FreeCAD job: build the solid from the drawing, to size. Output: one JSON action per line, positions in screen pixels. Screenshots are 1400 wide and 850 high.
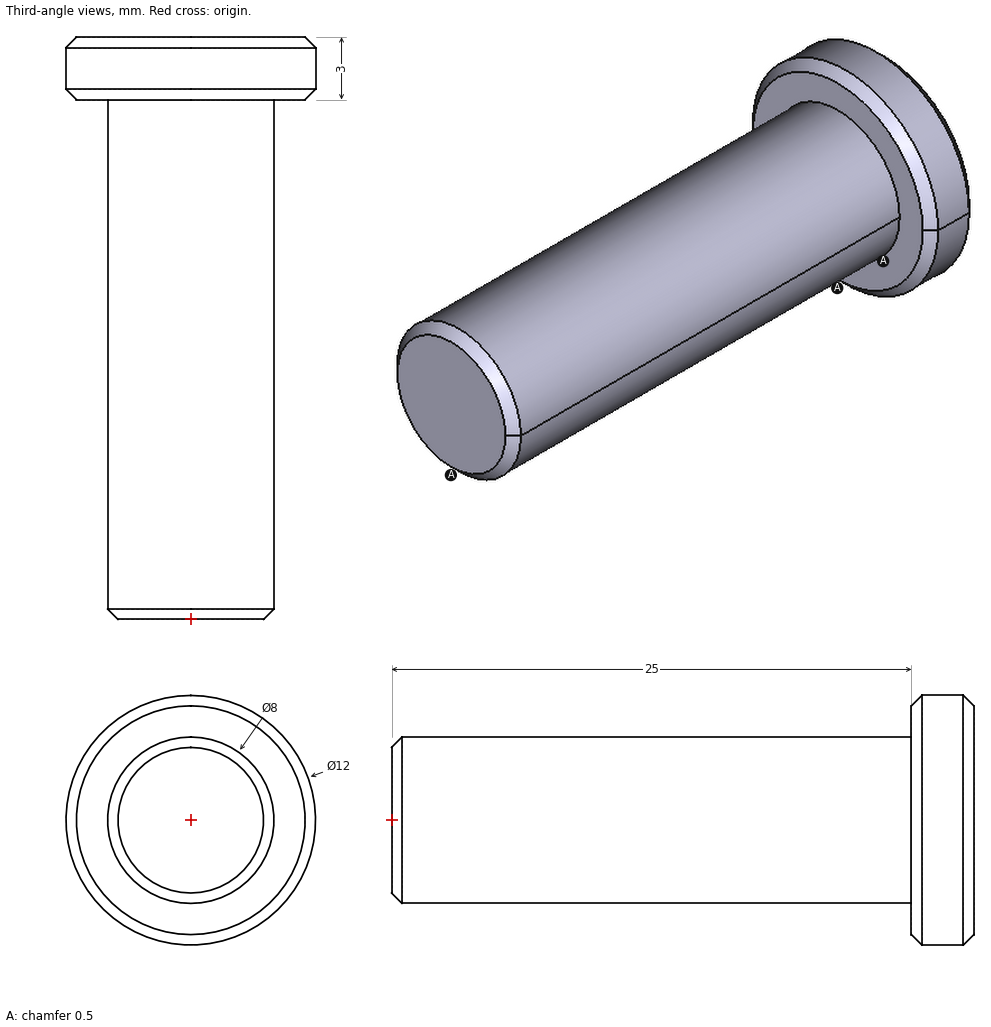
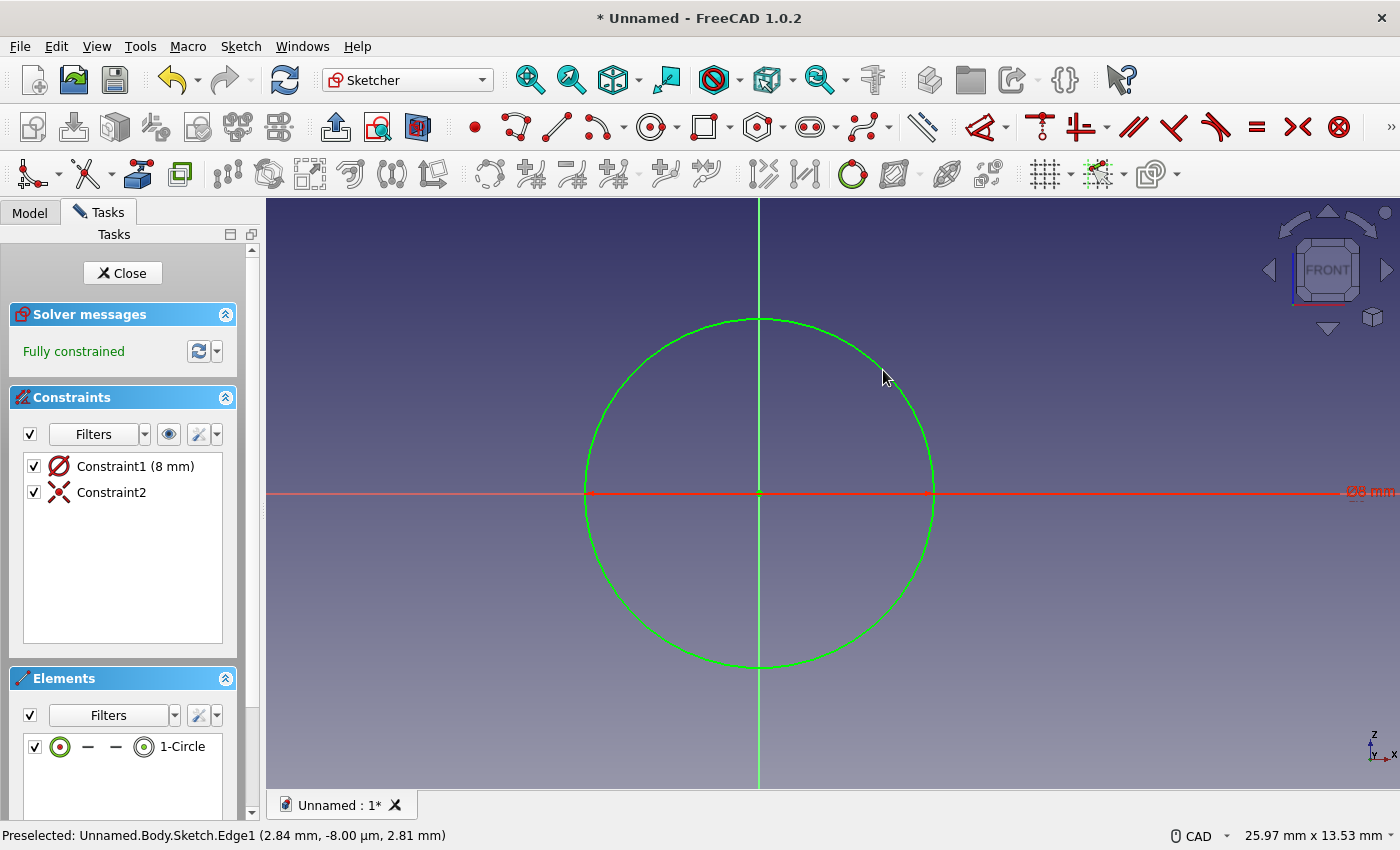
{"action": "left_click", "coordinate": [123, 273]}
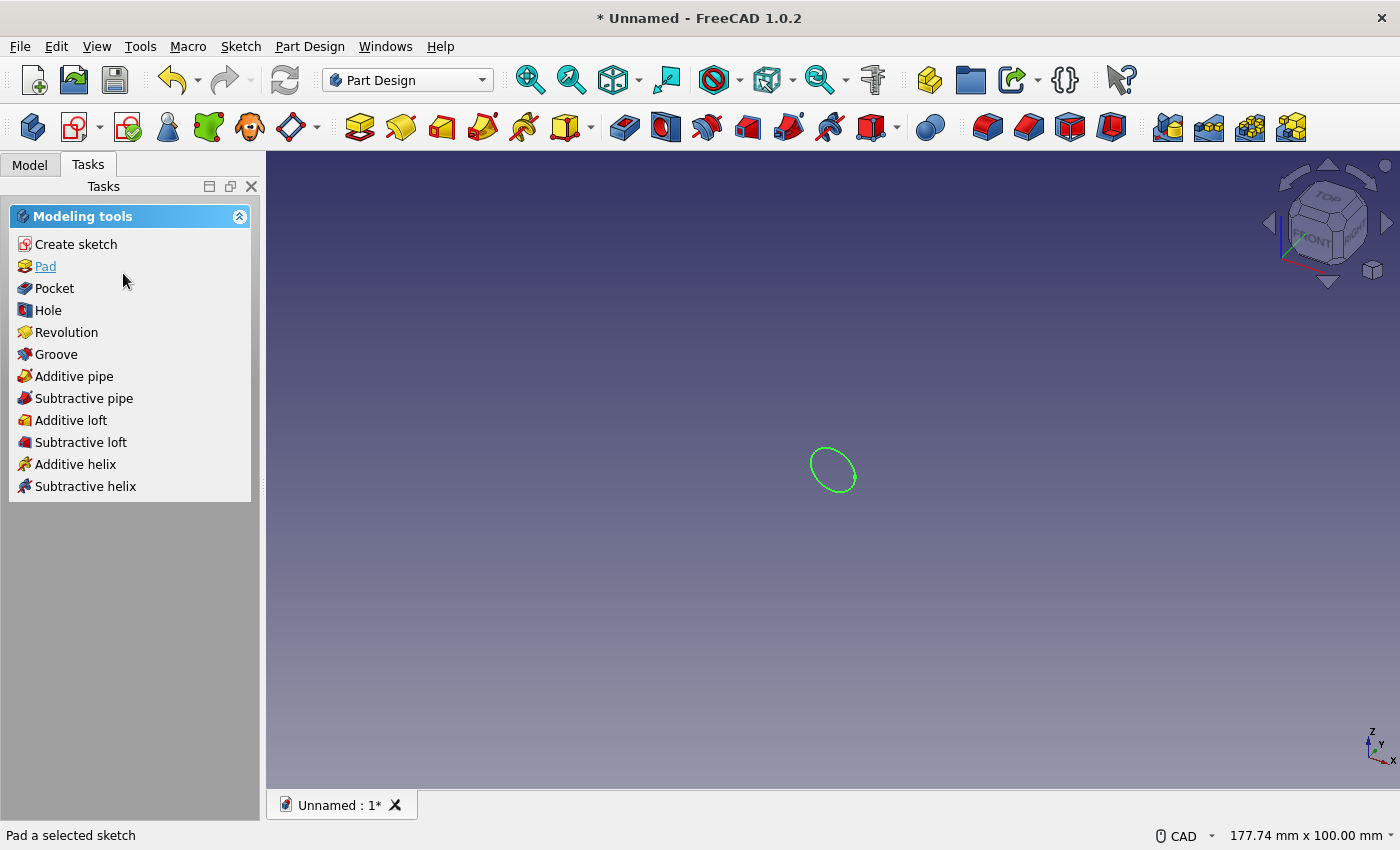
{"action": "left_click", "coordinate": [360, 128]}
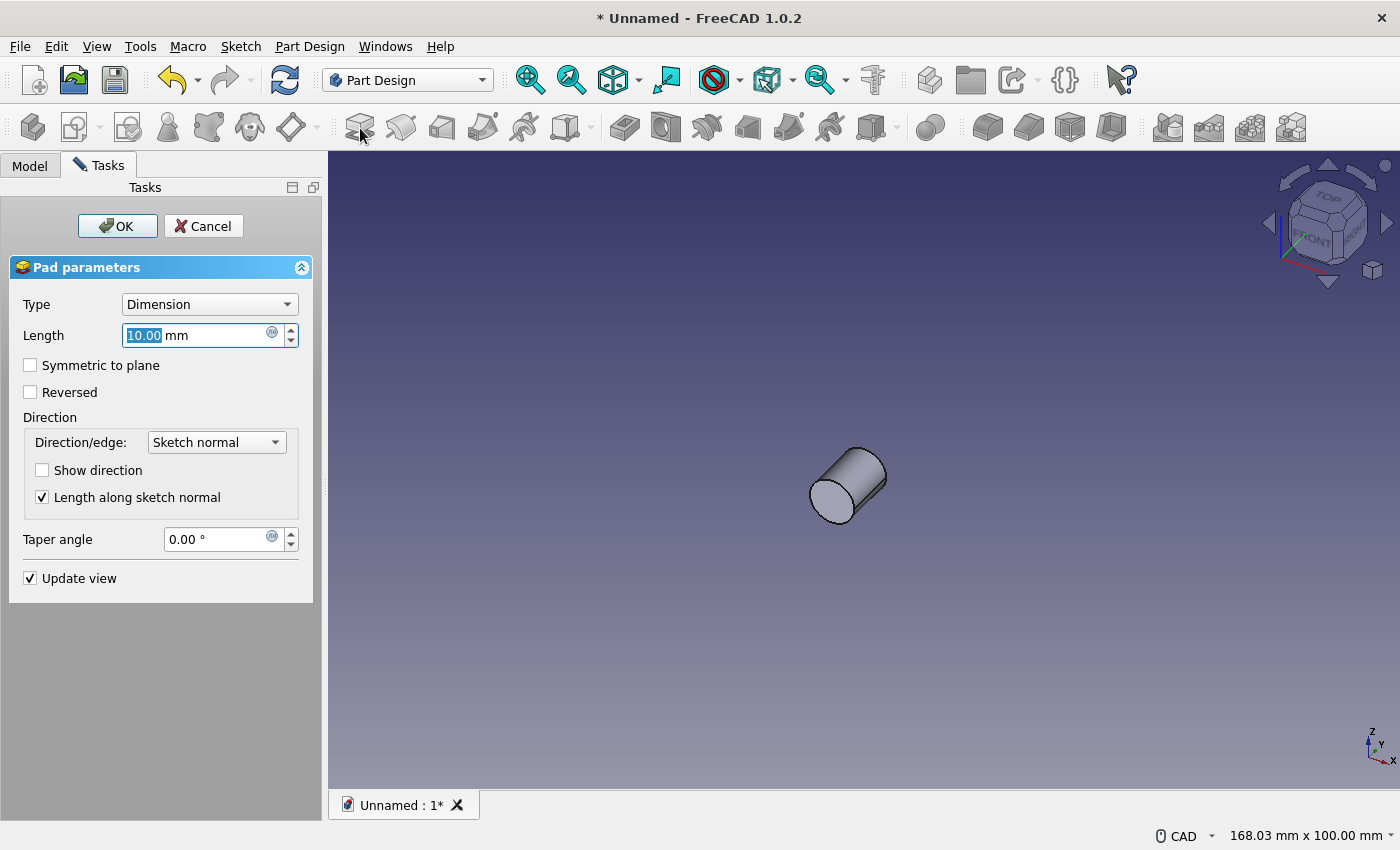
{"action": "type", "text": "25"}
{"action": "key", "text": "Tab"}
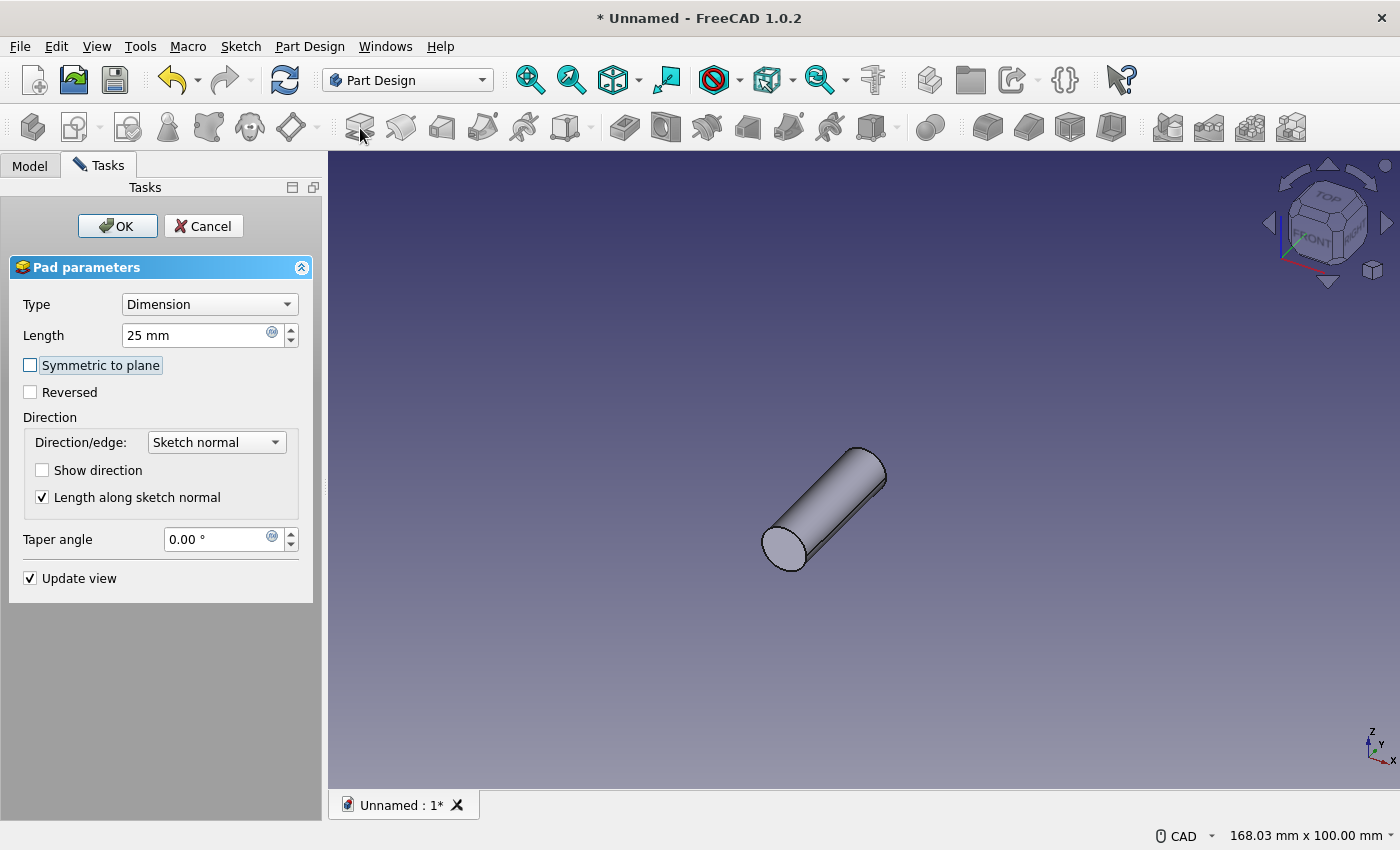
{"action": "left_click", "coordinate": [31, 392]}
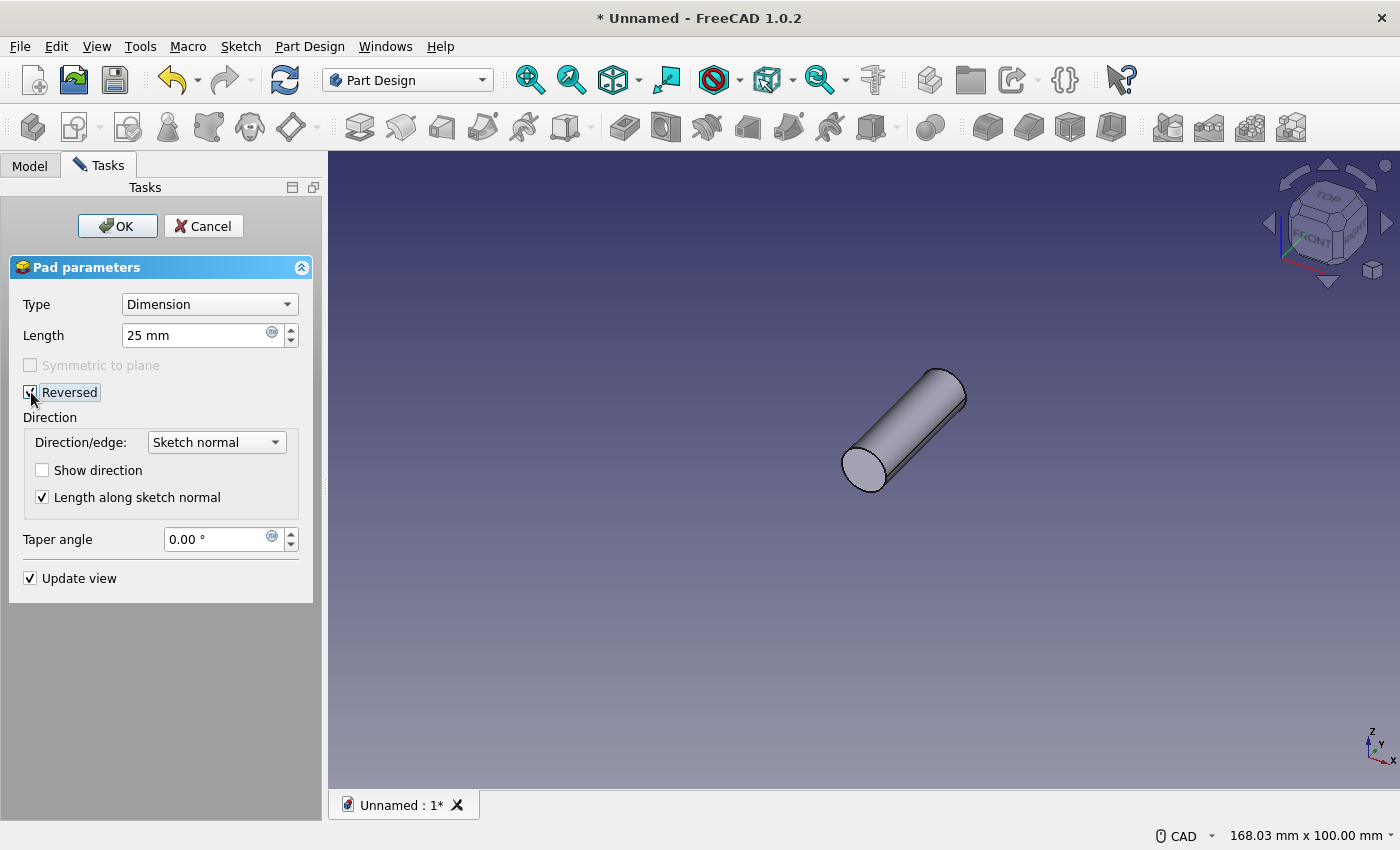
{"action": "left_click", "coordinate": [118, 226]}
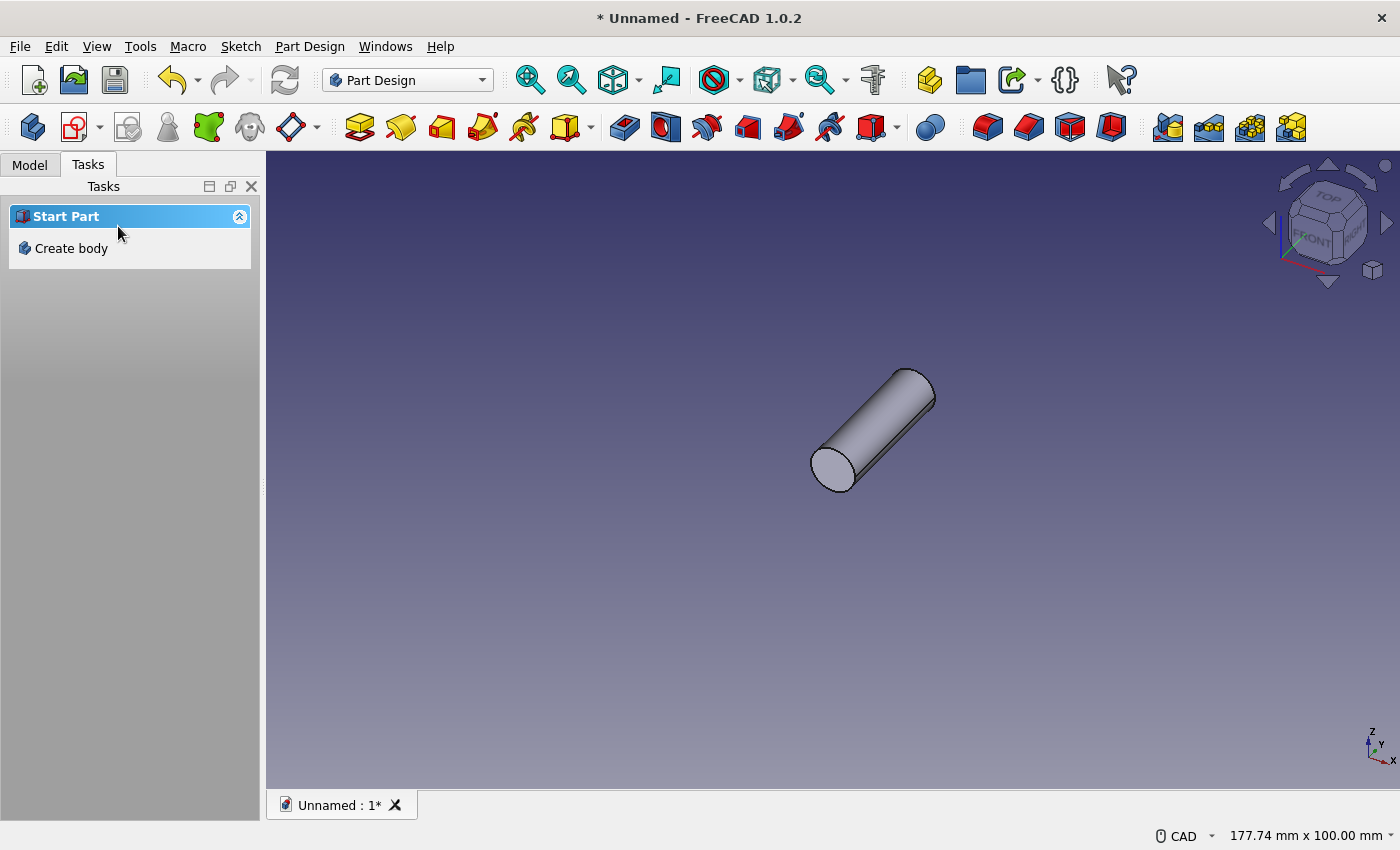
{"action": "left_click", "coordinate": [531, 80]}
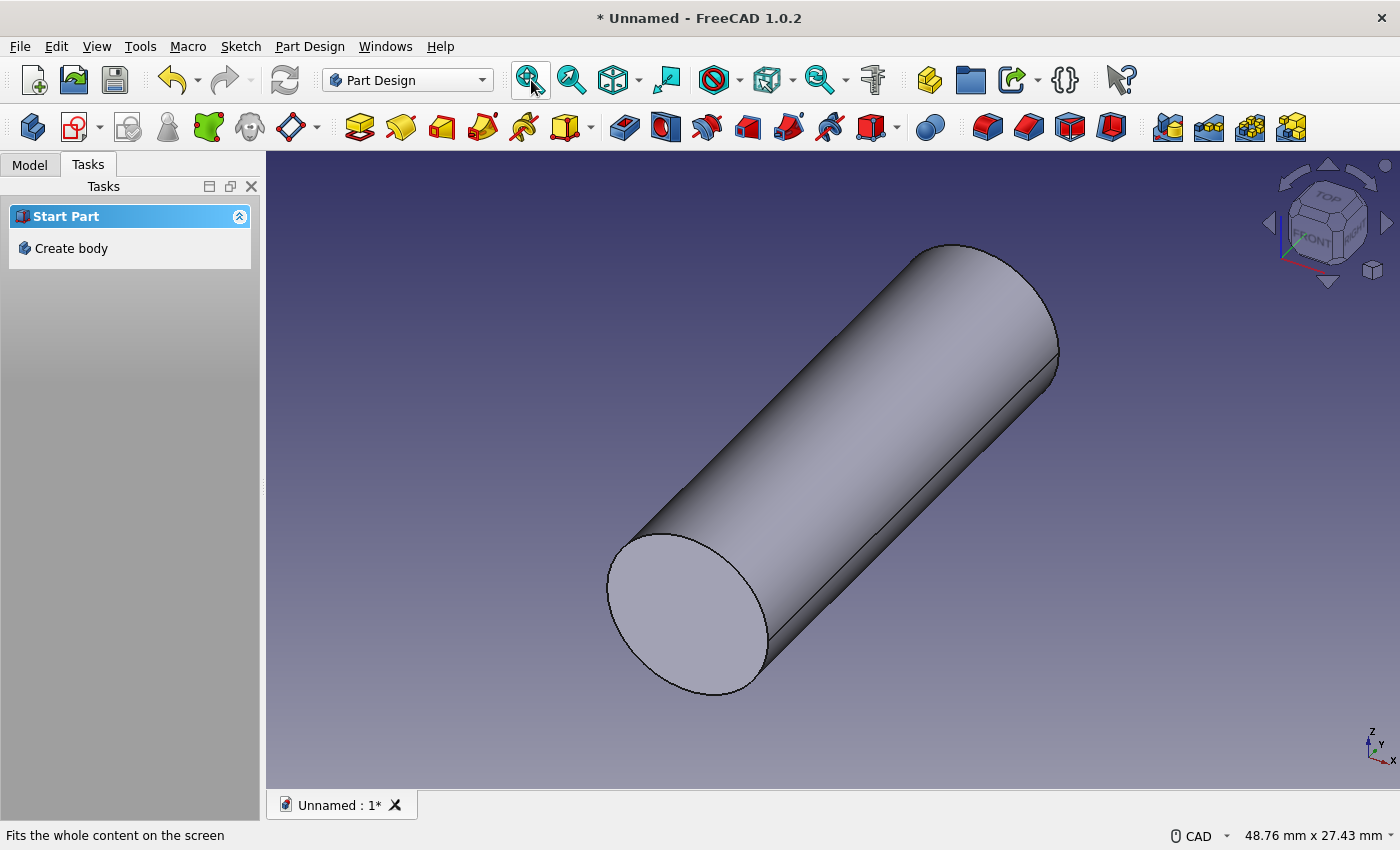
{"action": "key", "text": "4"}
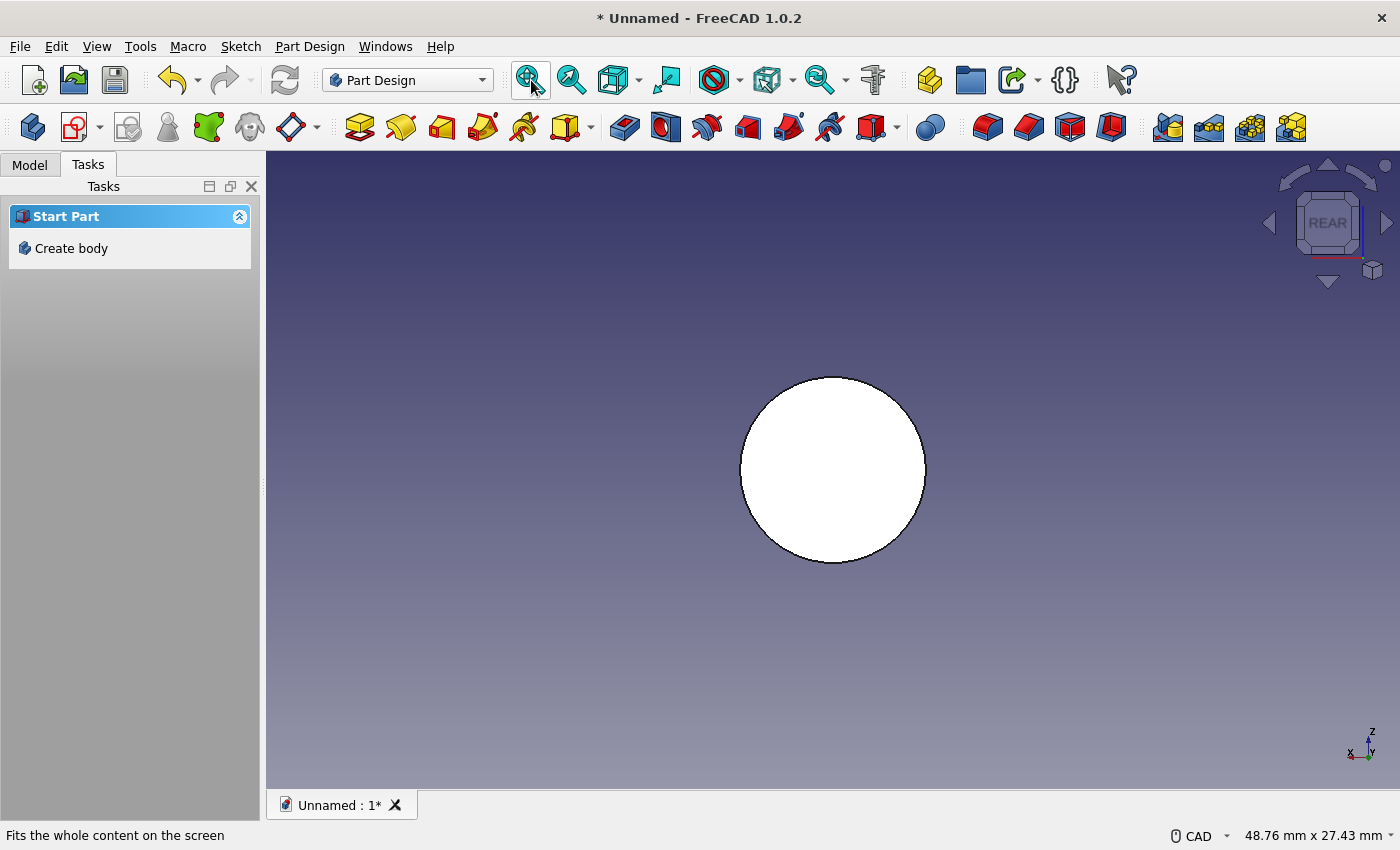
{"action": "left_click", "coordinate": [531, 80]}